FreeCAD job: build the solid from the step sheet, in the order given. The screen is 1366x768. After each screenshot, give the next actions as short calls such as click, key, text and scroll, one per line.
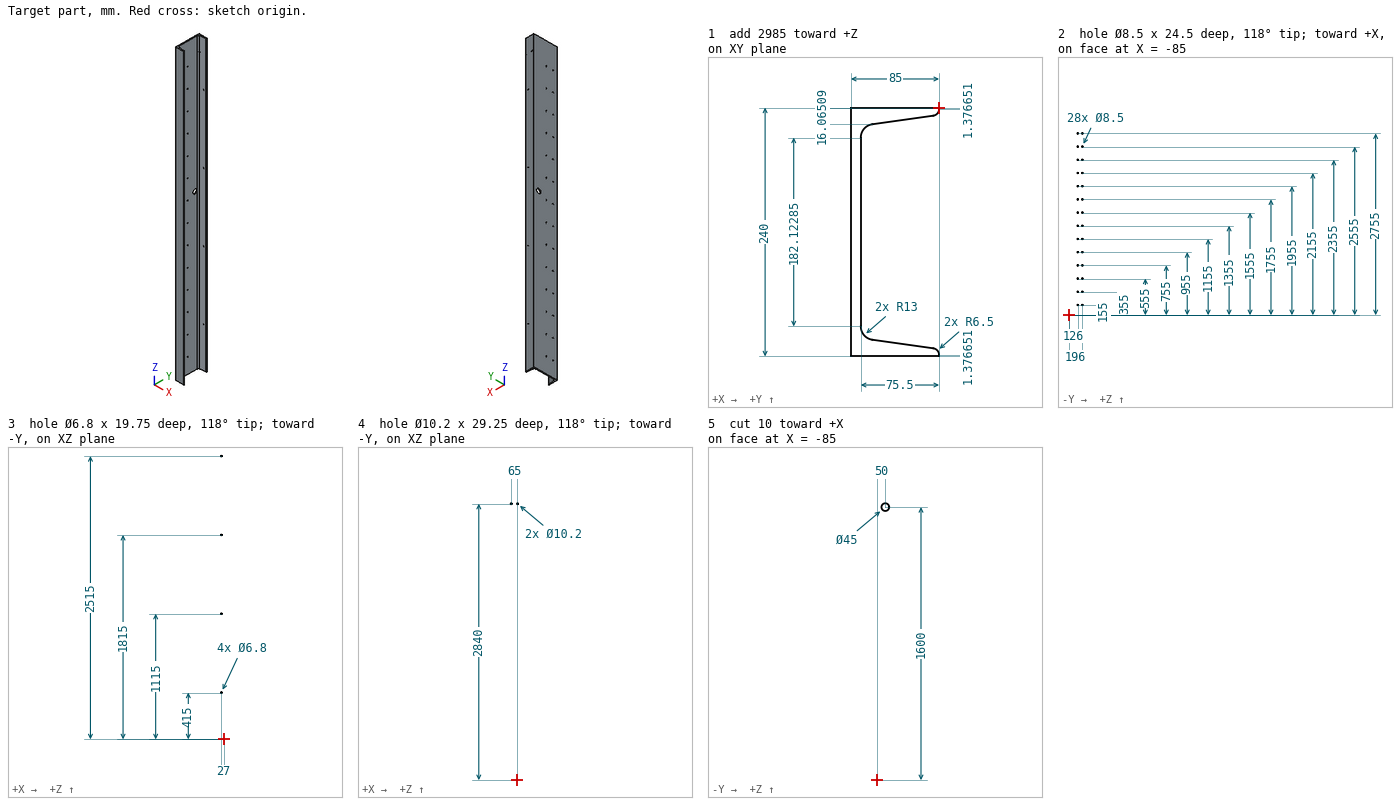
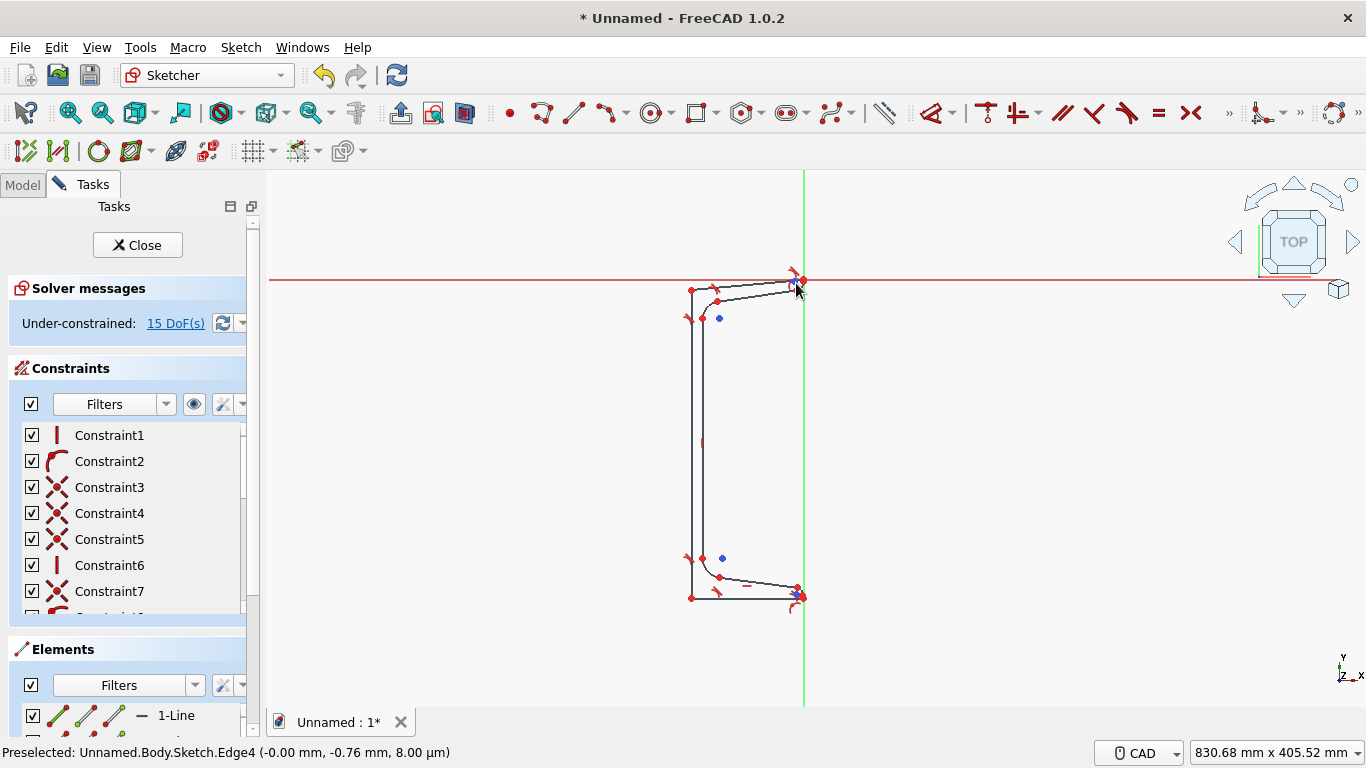
scroll(800, 289, up, 7)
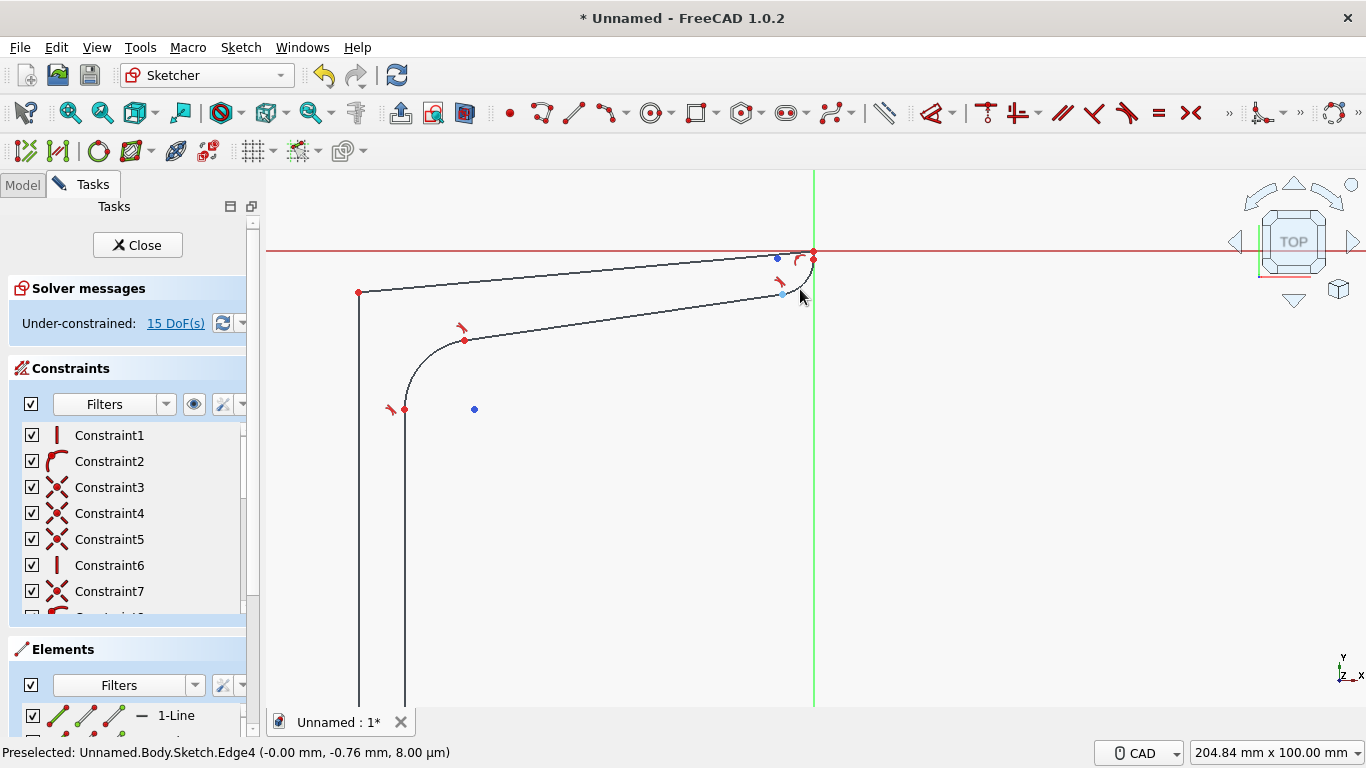
click(797, 289)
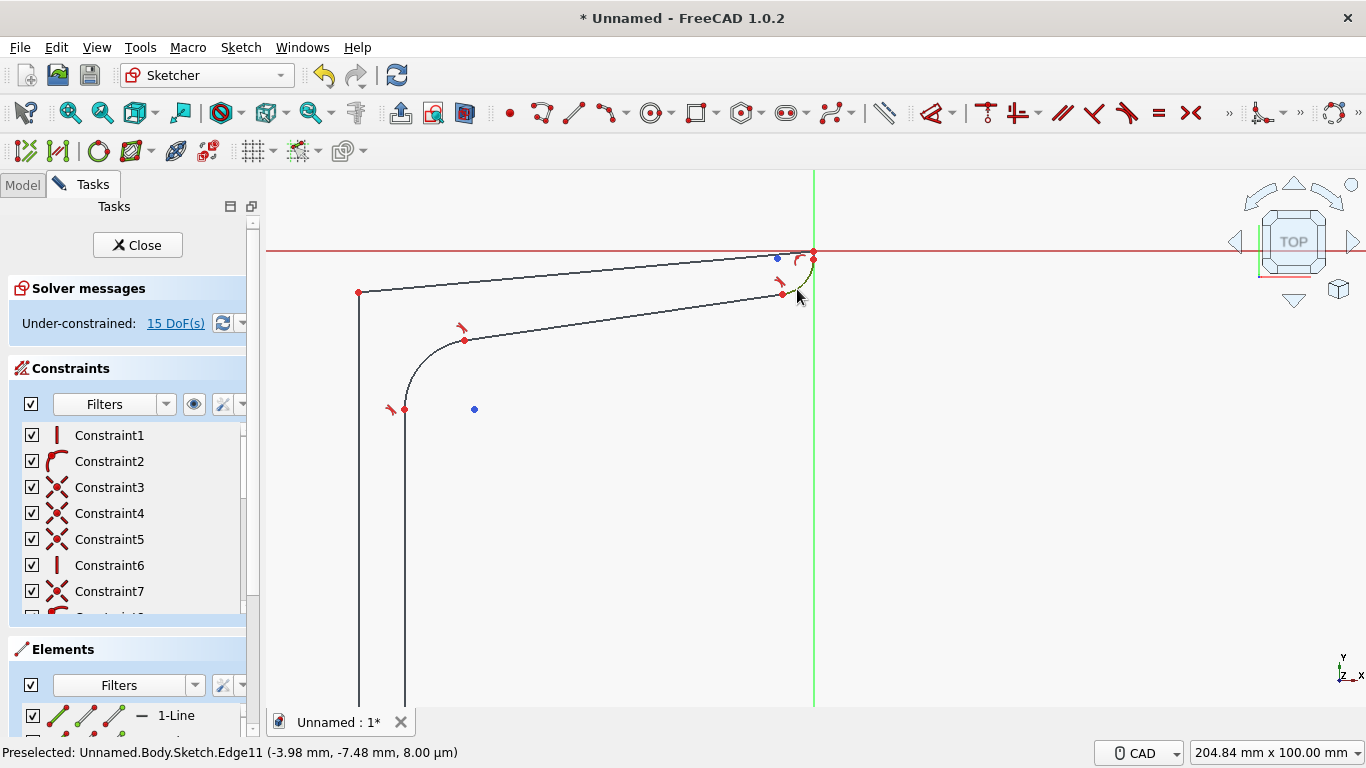
click(1128, 114)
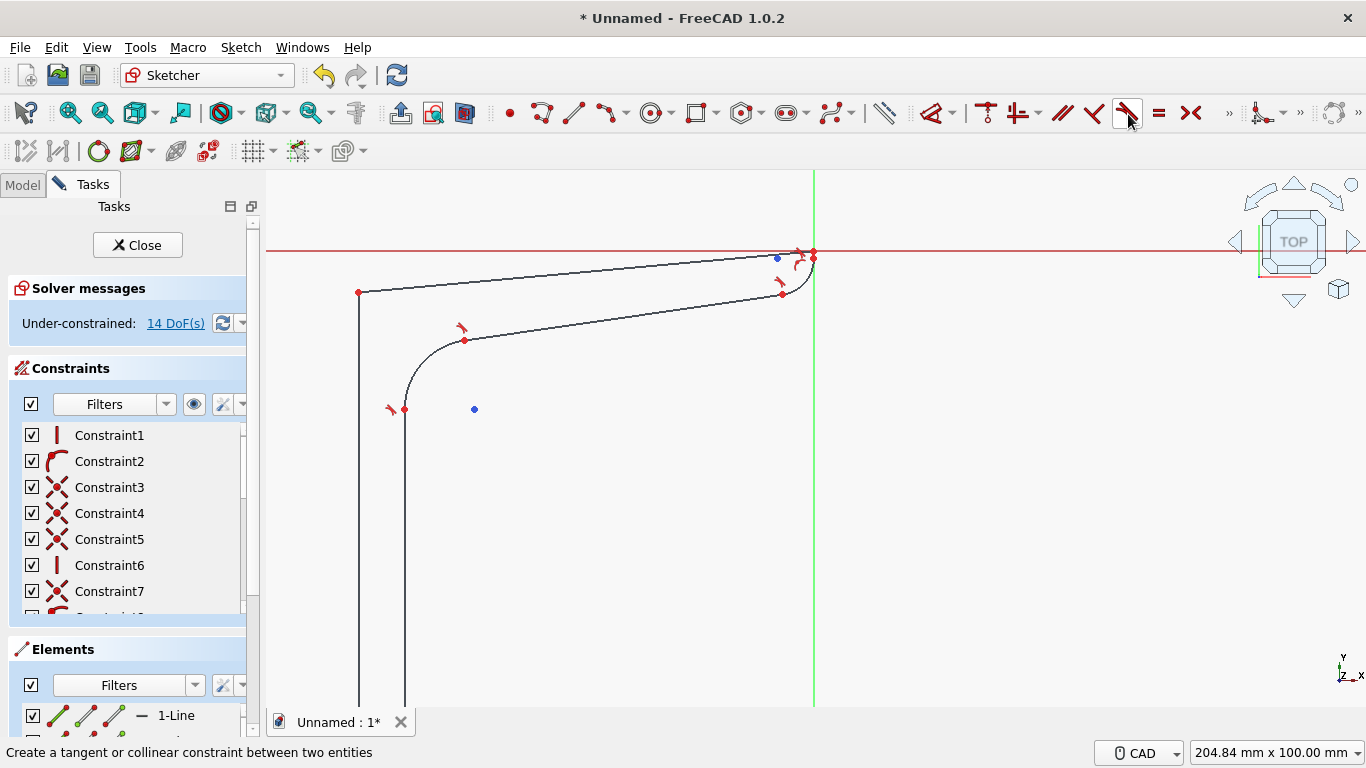
scroll(800, 289, down, 7)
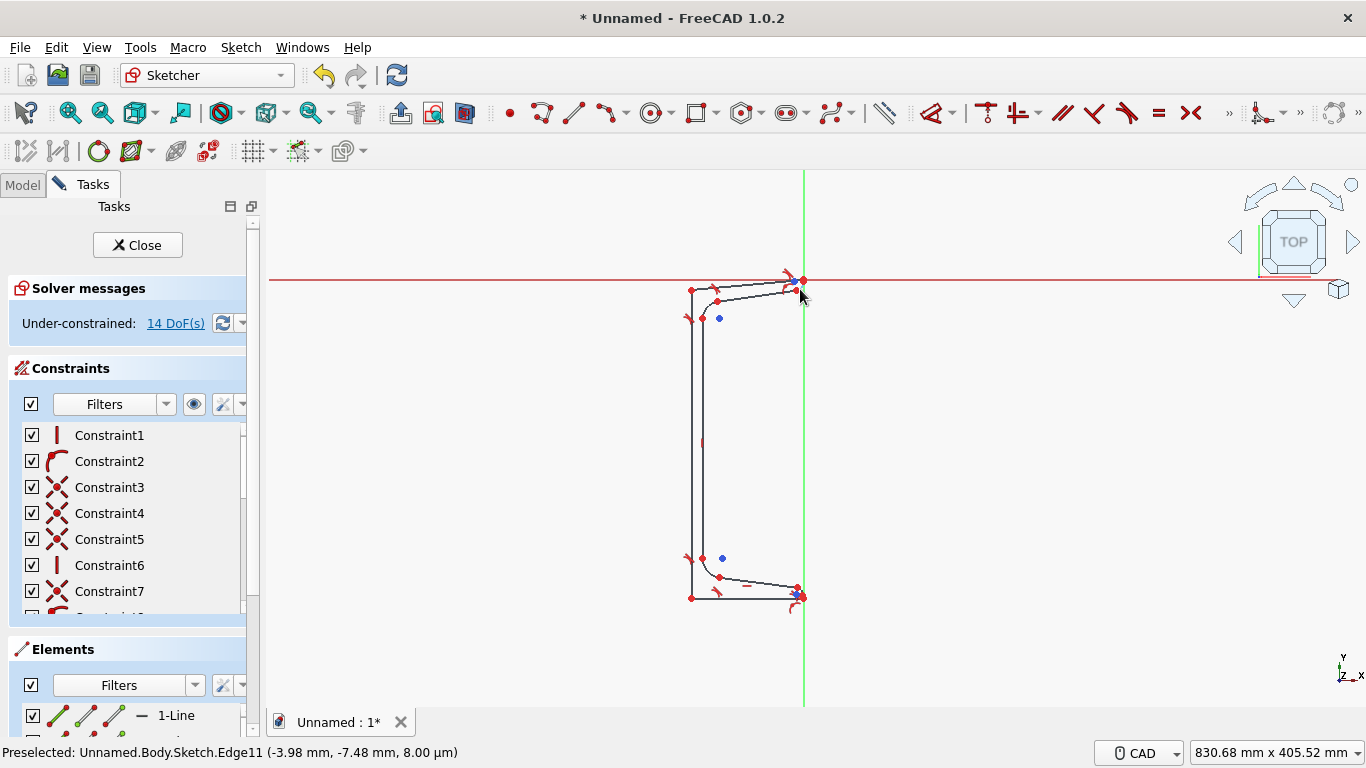
scroll(803, 597, up, 12)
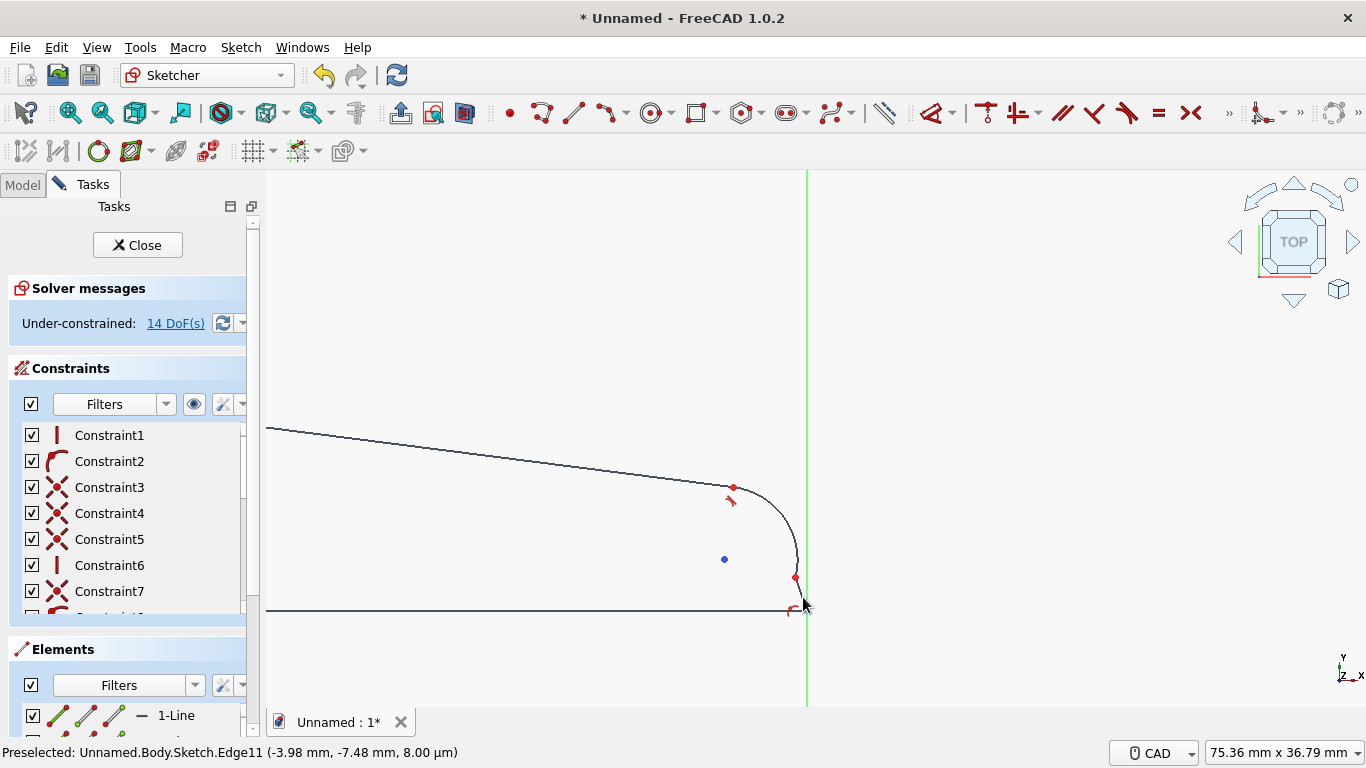
click(801, 594)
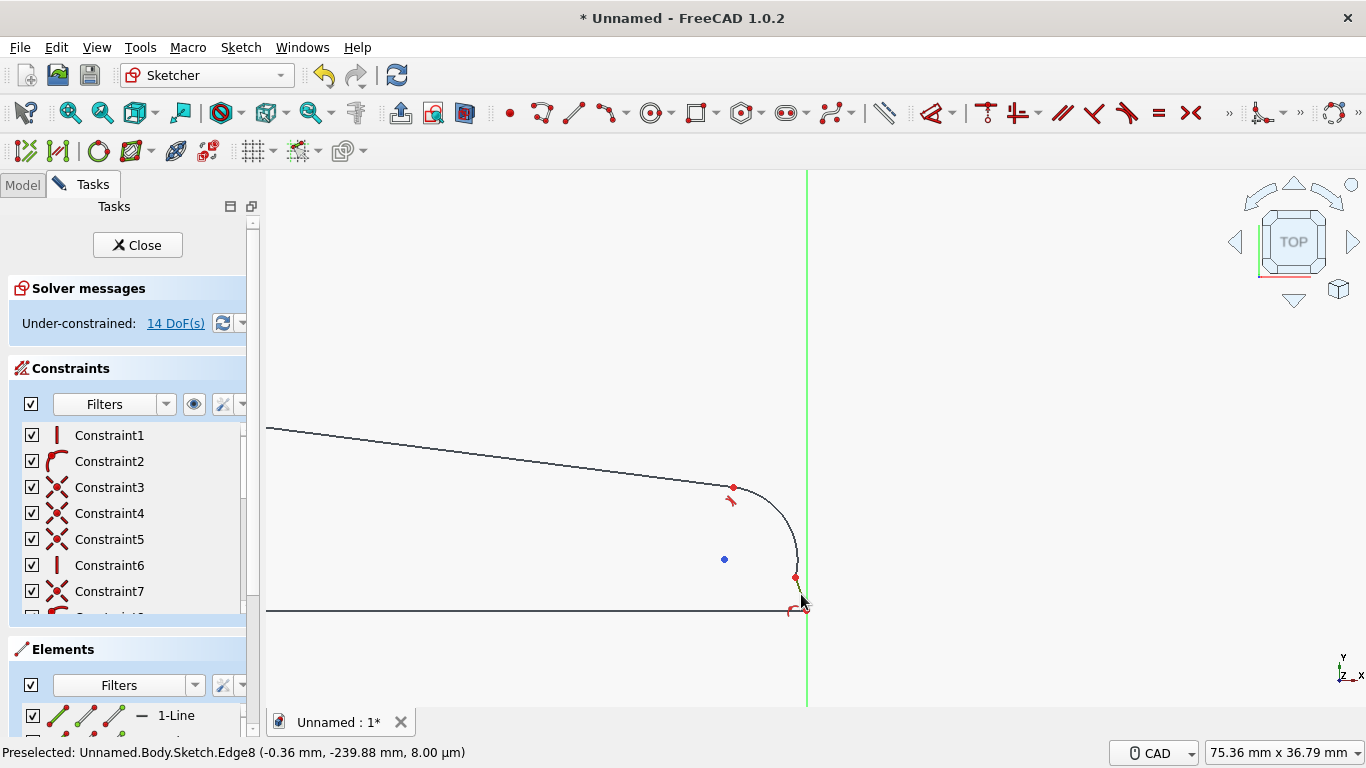
click(795, 541)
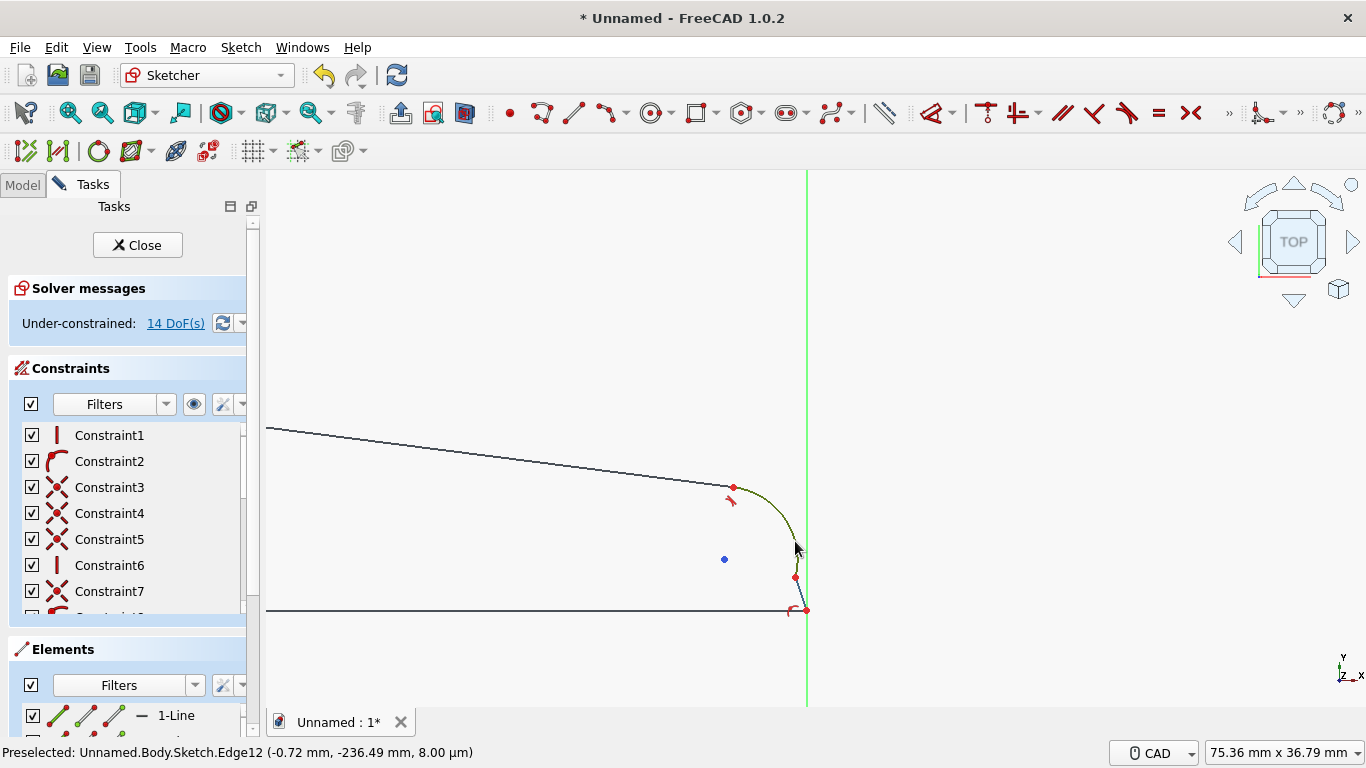
click(1128, 114)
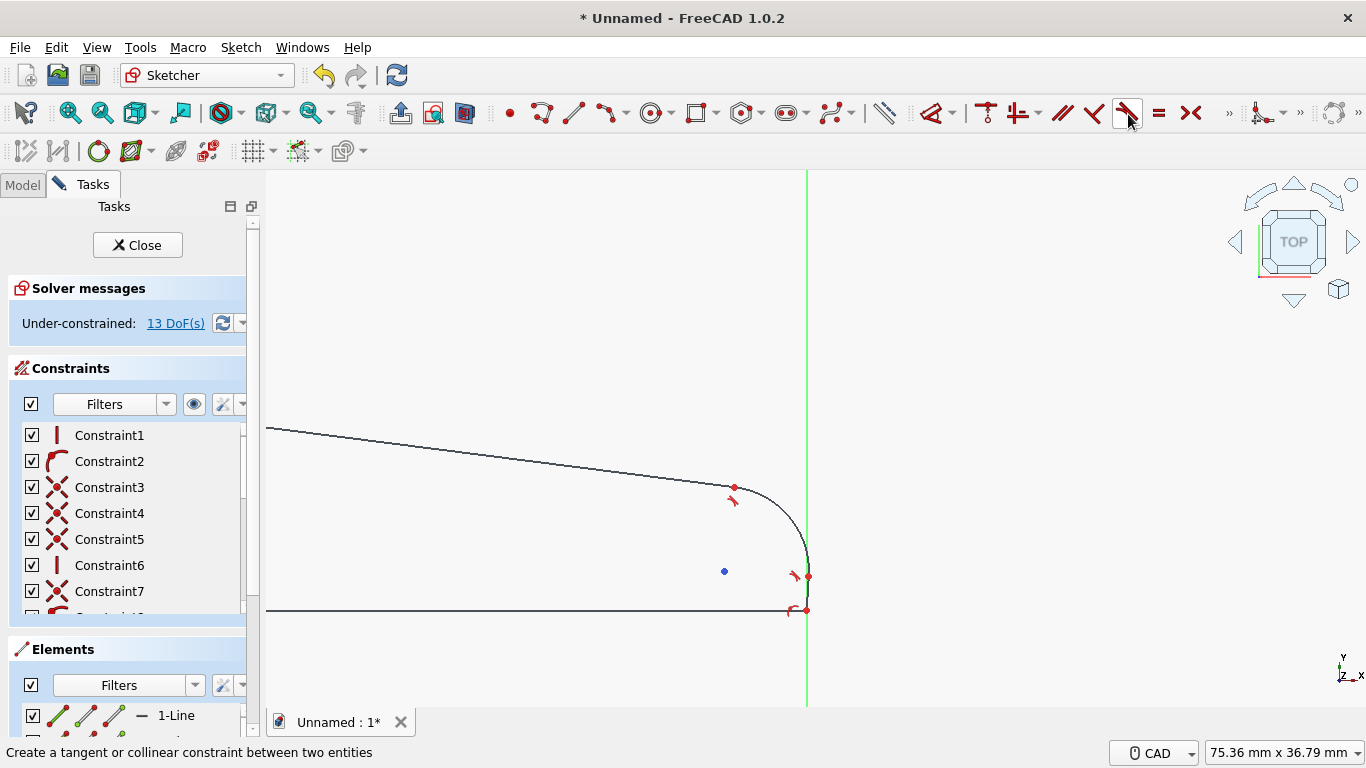
scroll(803, 597, down, 12)